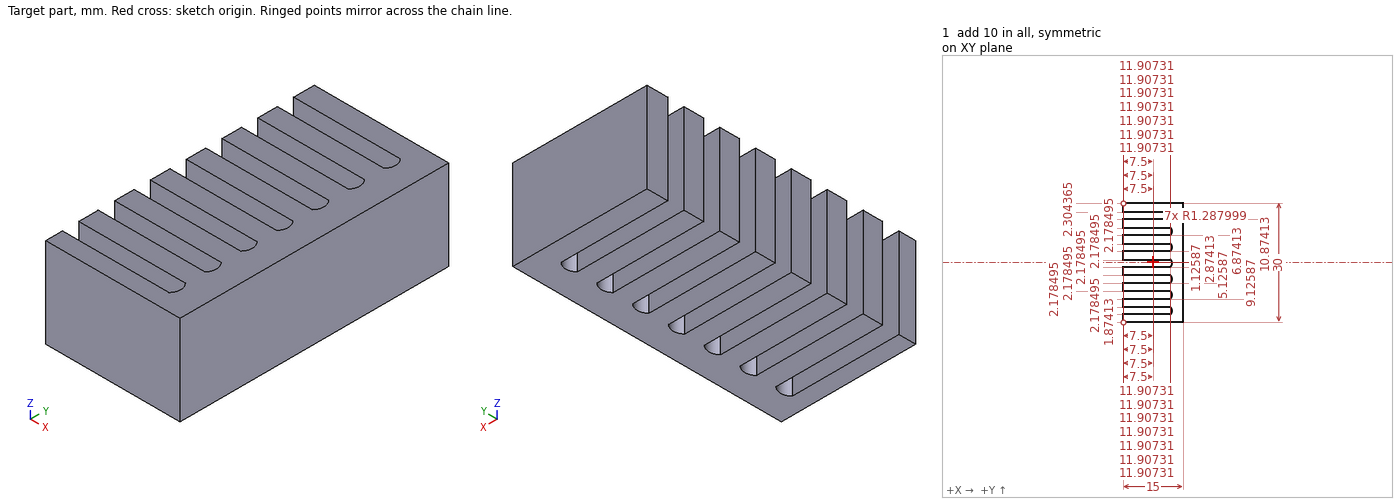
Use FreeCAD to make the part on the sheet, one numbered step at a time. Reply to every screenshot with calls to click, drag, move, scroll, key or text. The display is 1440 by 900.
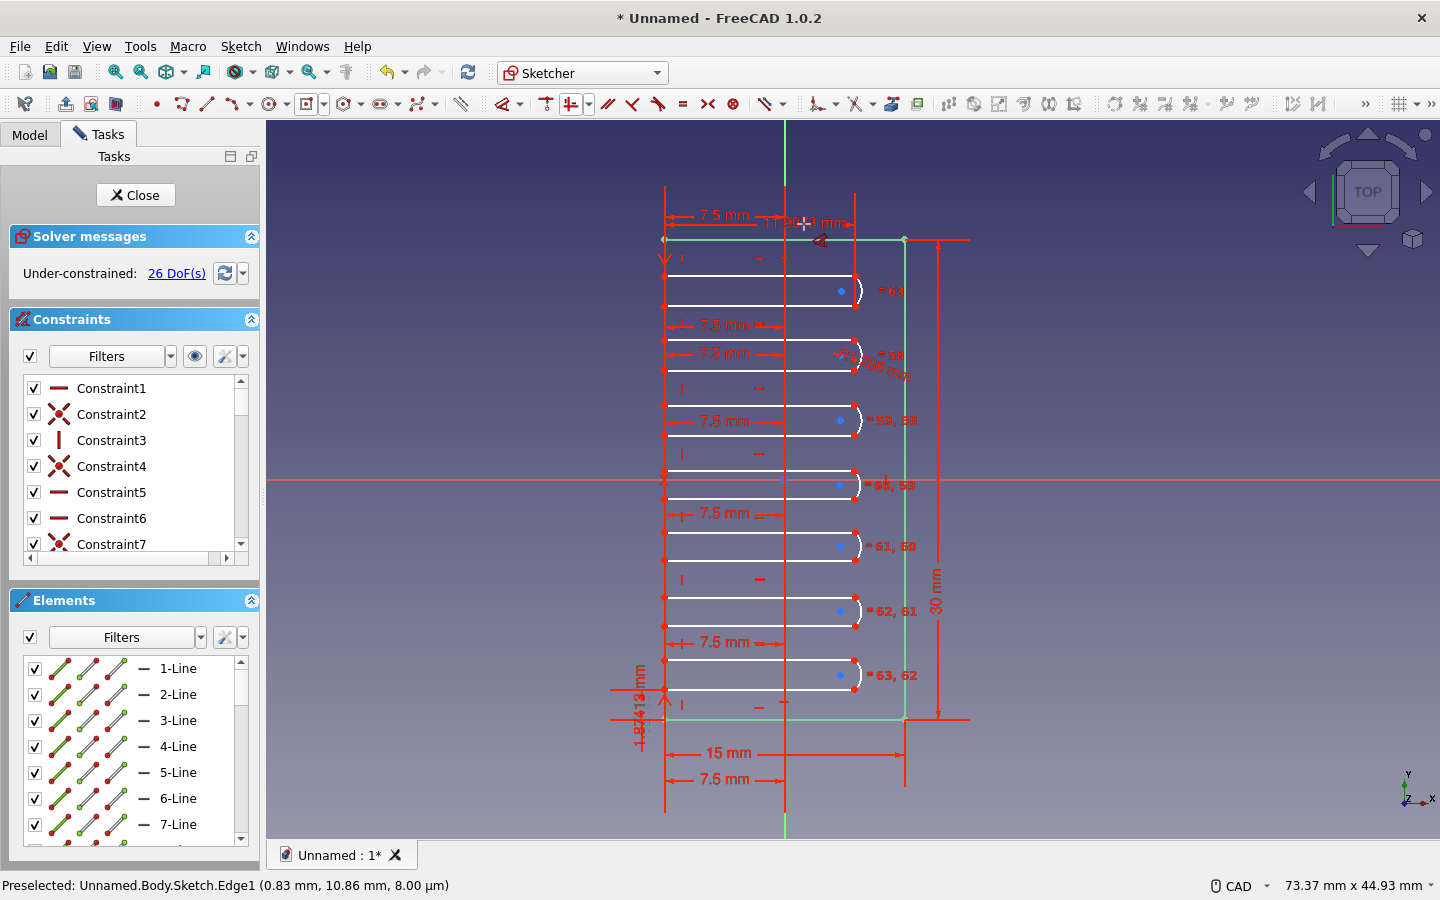
scroll(665, 316, up, 2)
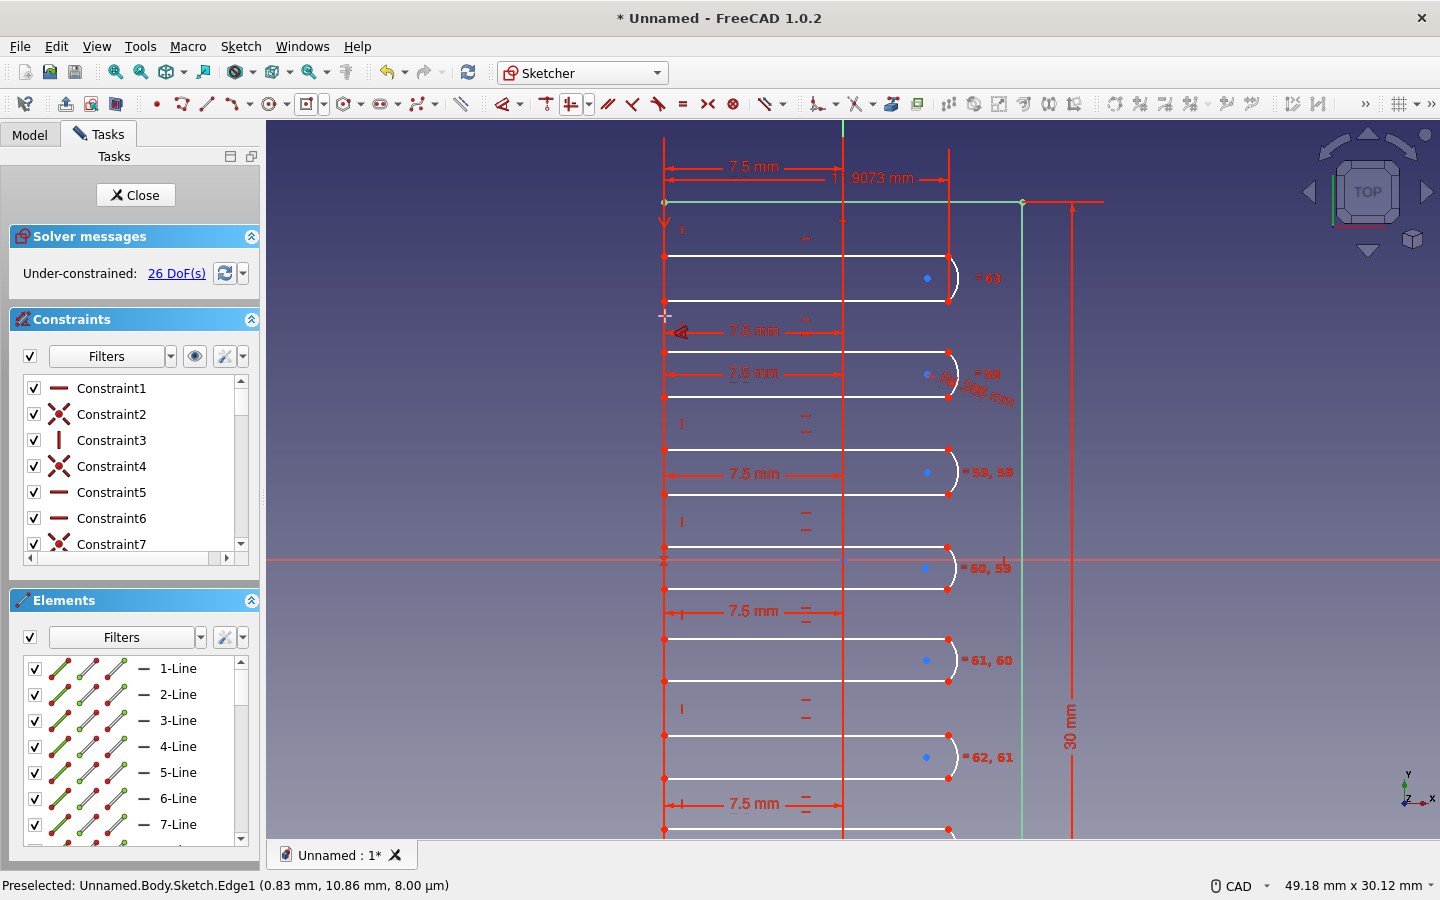
click(664, 316)
click(630, 327)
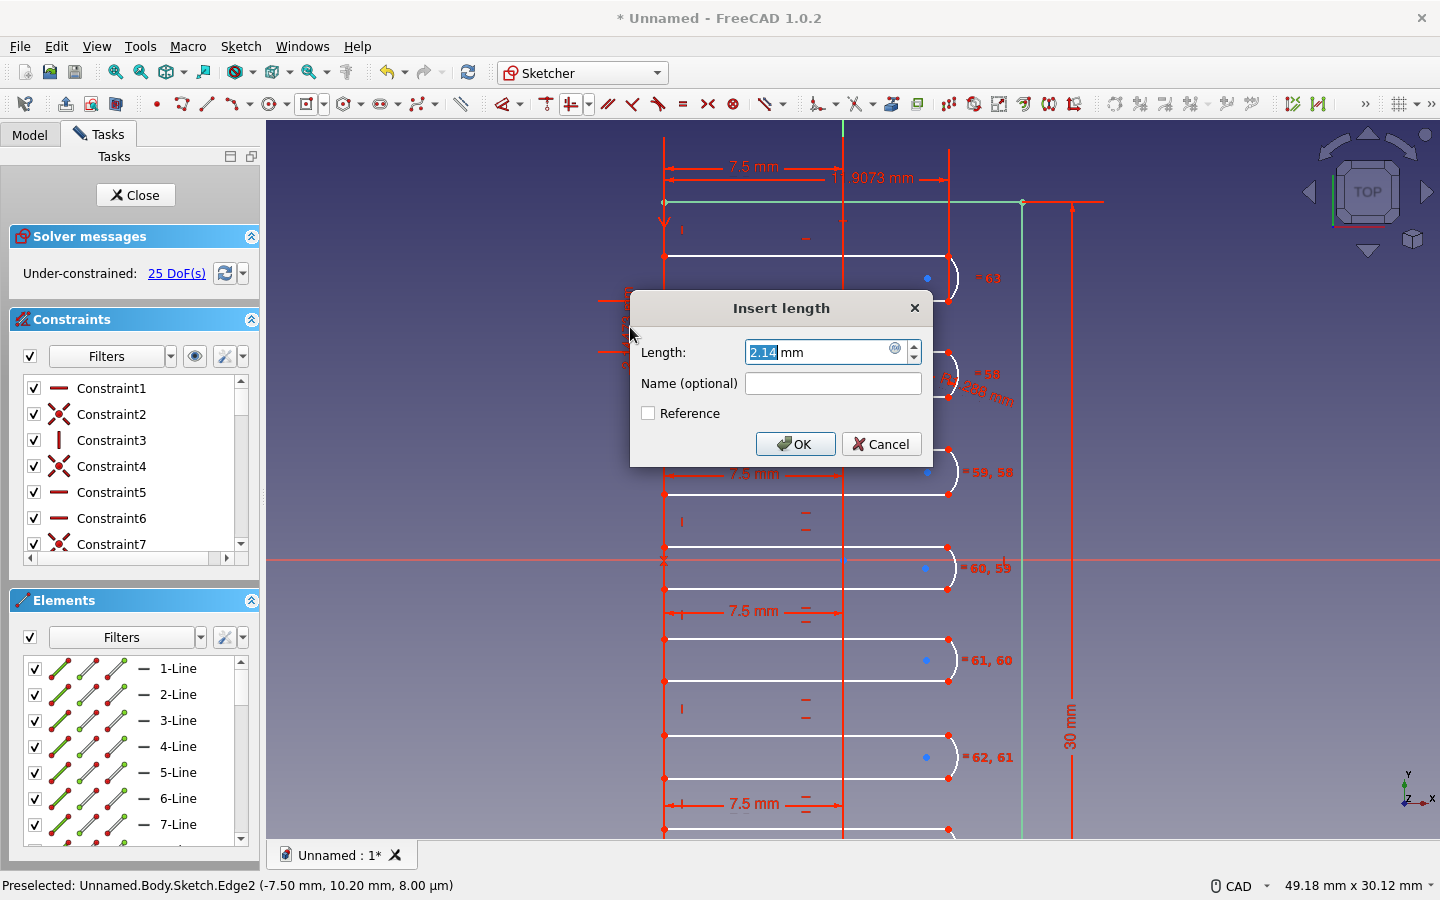
text(2.178495)
key(Return)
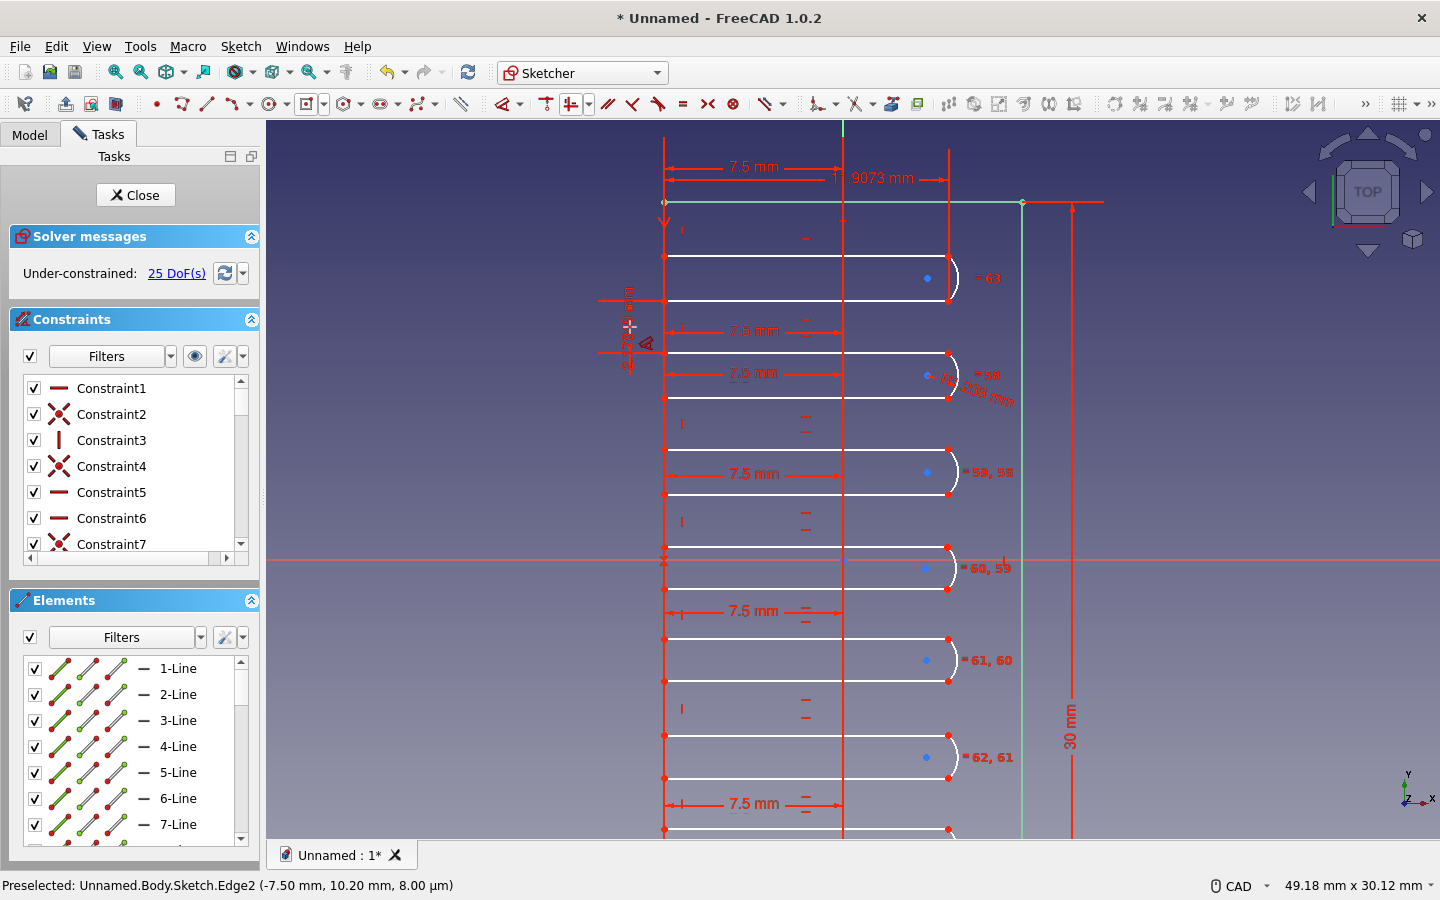
click(750, 353)
click(872, 319)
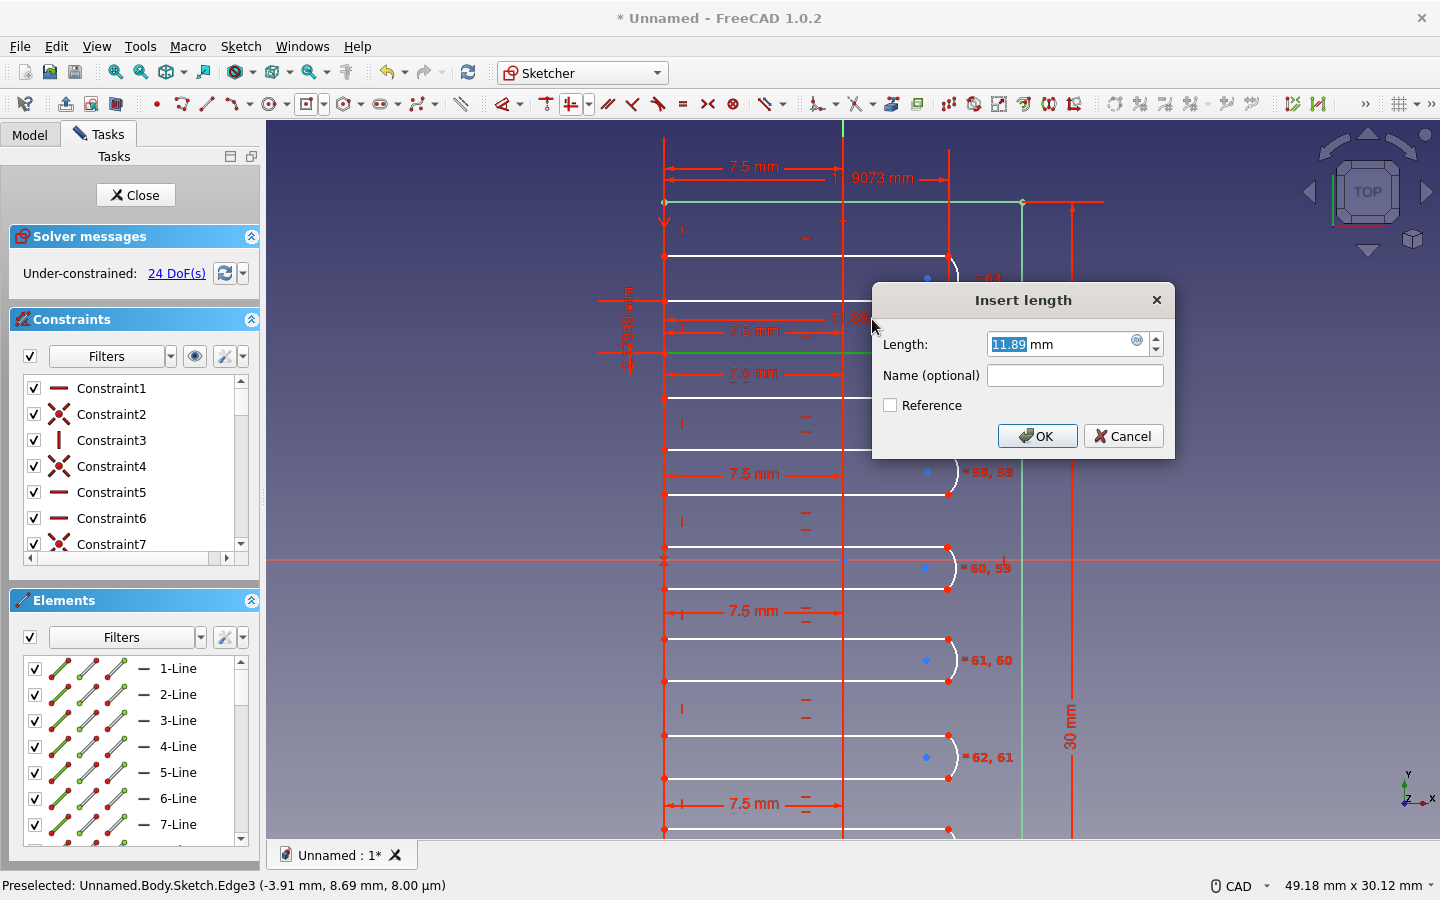
text(11.90731)
key(Return)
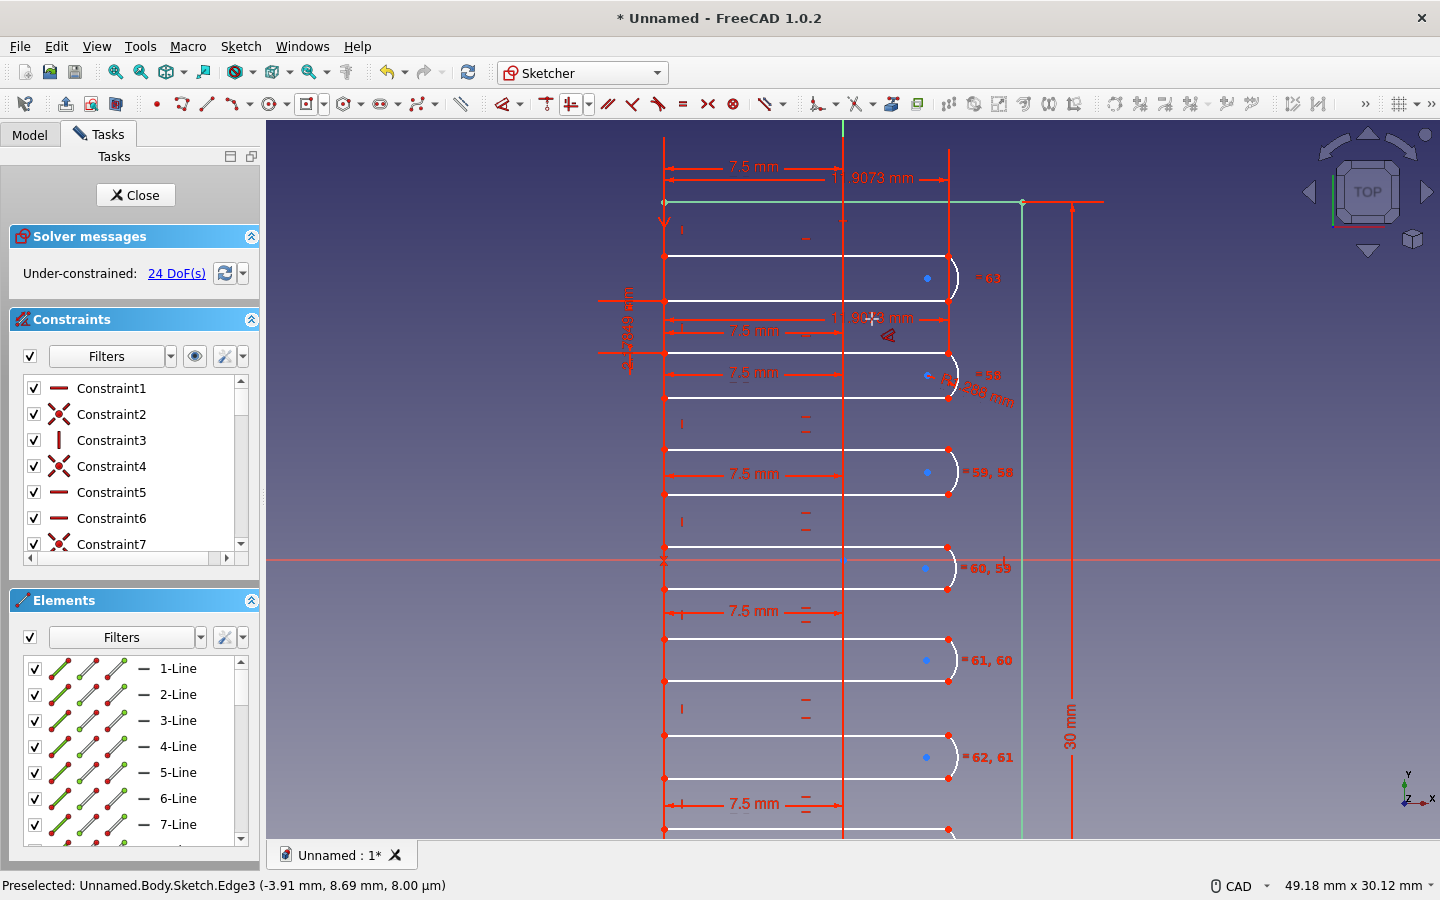
click(863, 398)
click(806, 432)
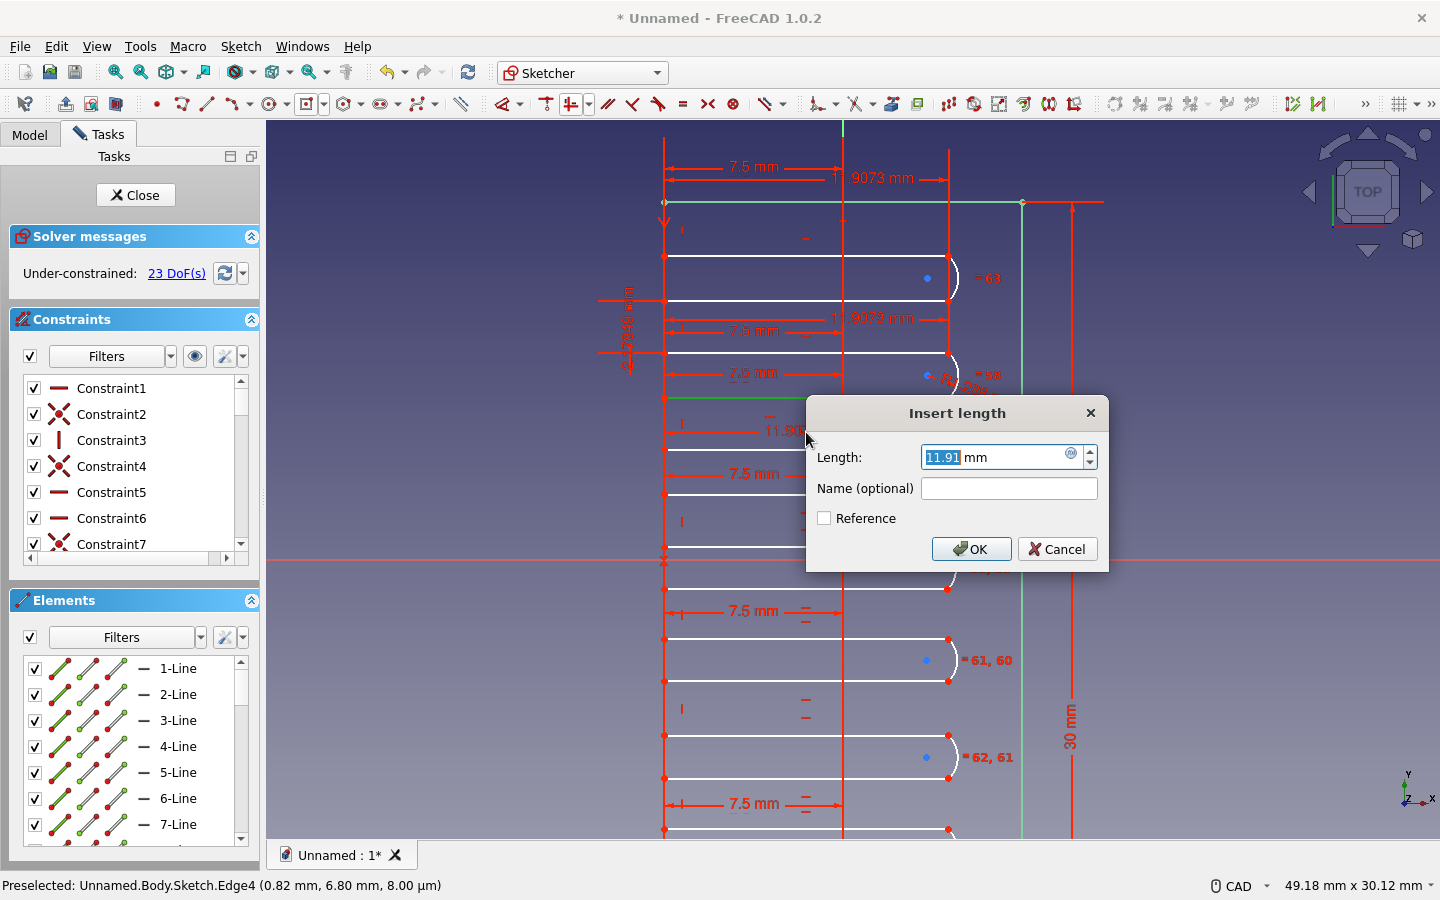
text(11.90731)
key(Return)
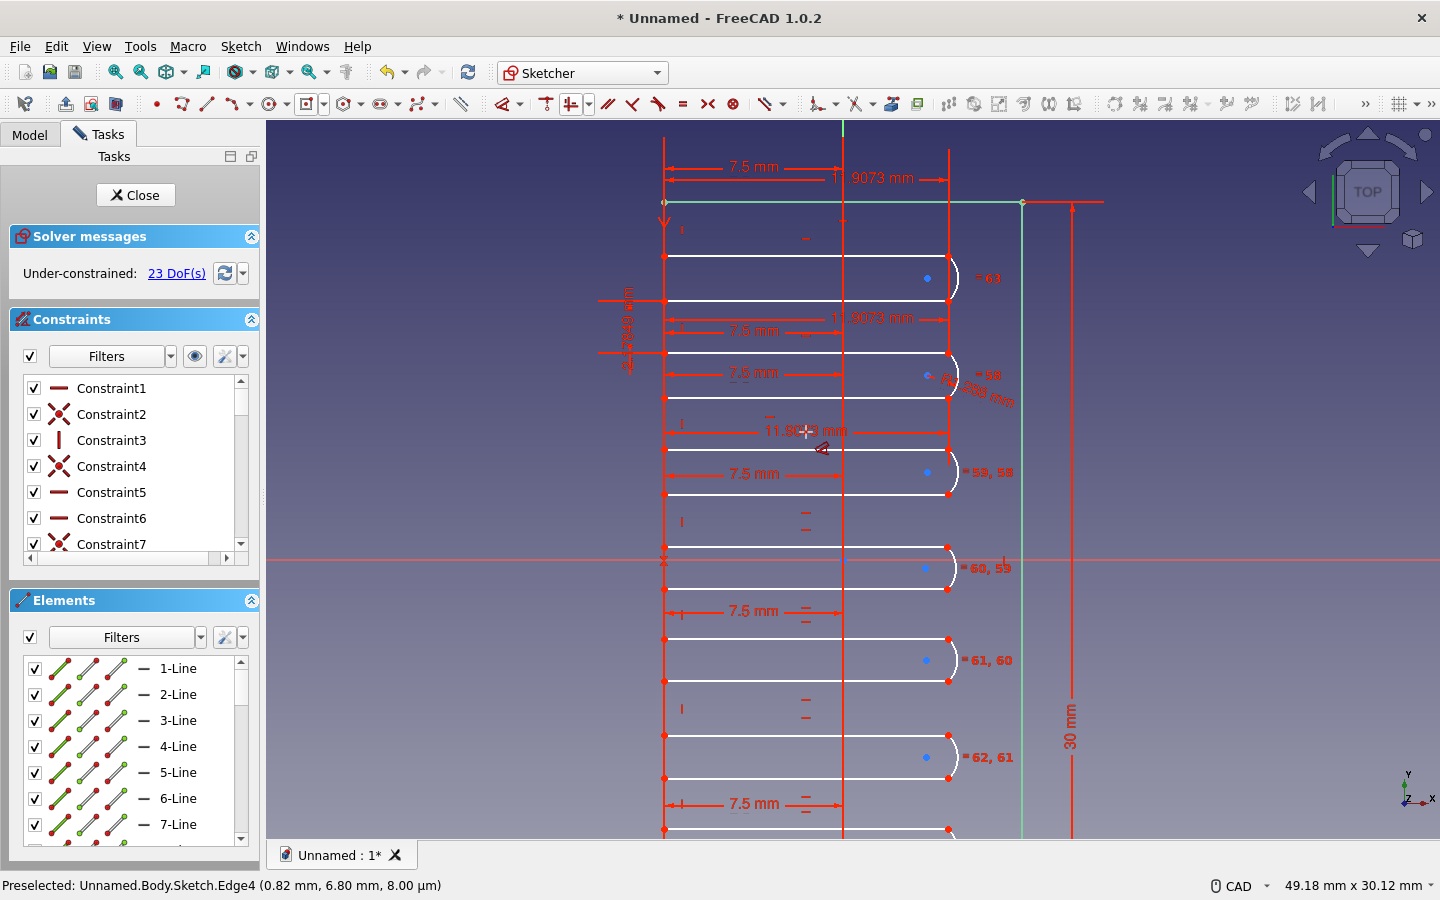
click(664, 414)
click(630, 424)